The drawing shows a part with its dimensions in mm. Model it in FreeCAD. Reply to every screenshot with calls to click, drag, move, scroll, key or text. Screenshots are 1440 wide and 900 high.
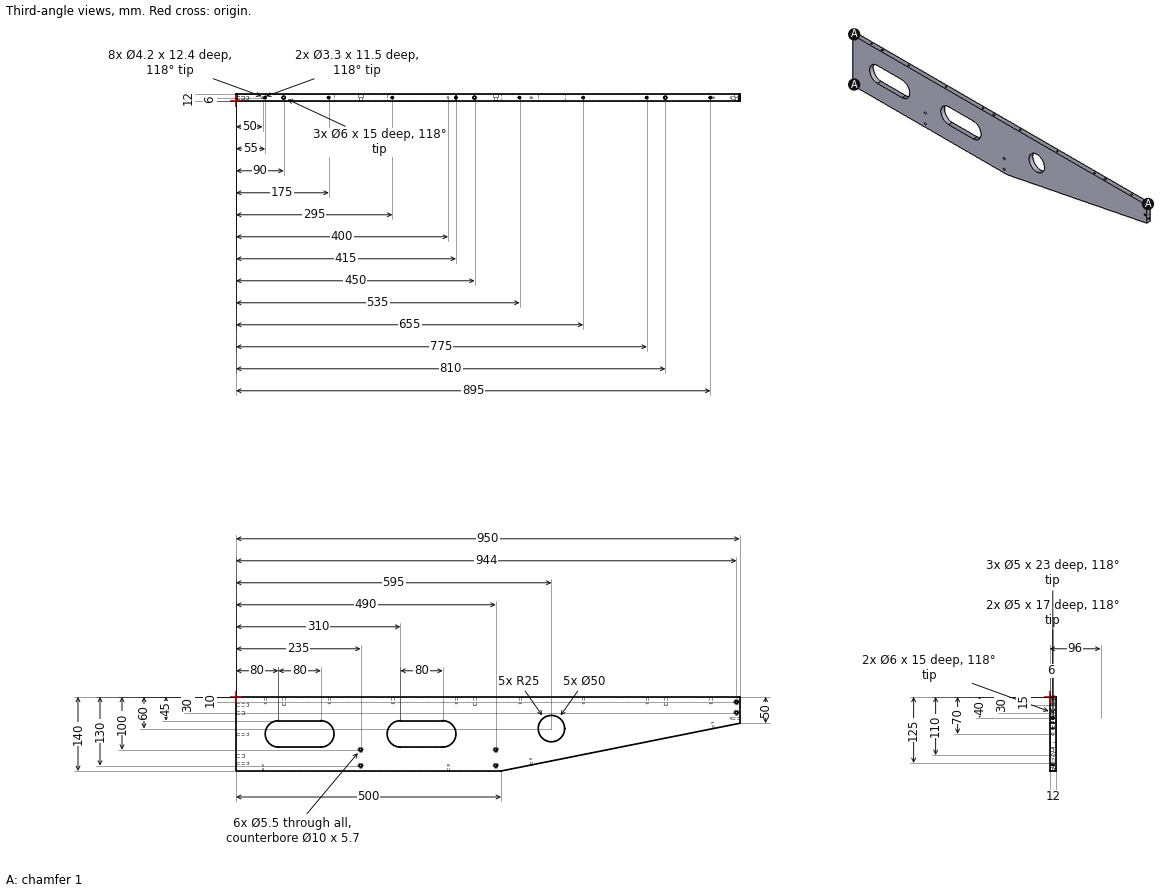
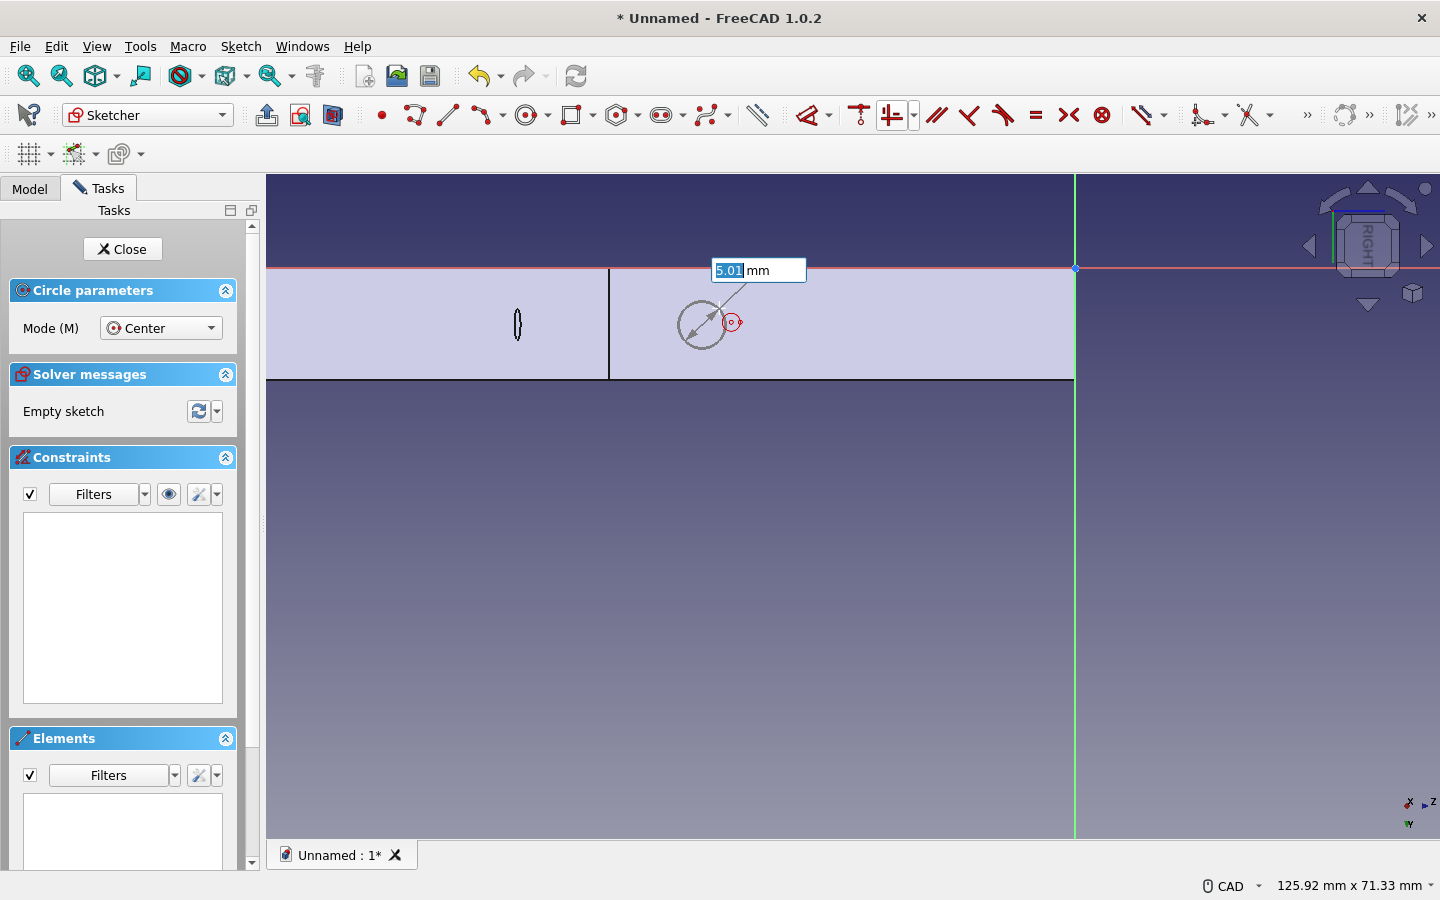
text(5)
key(Return)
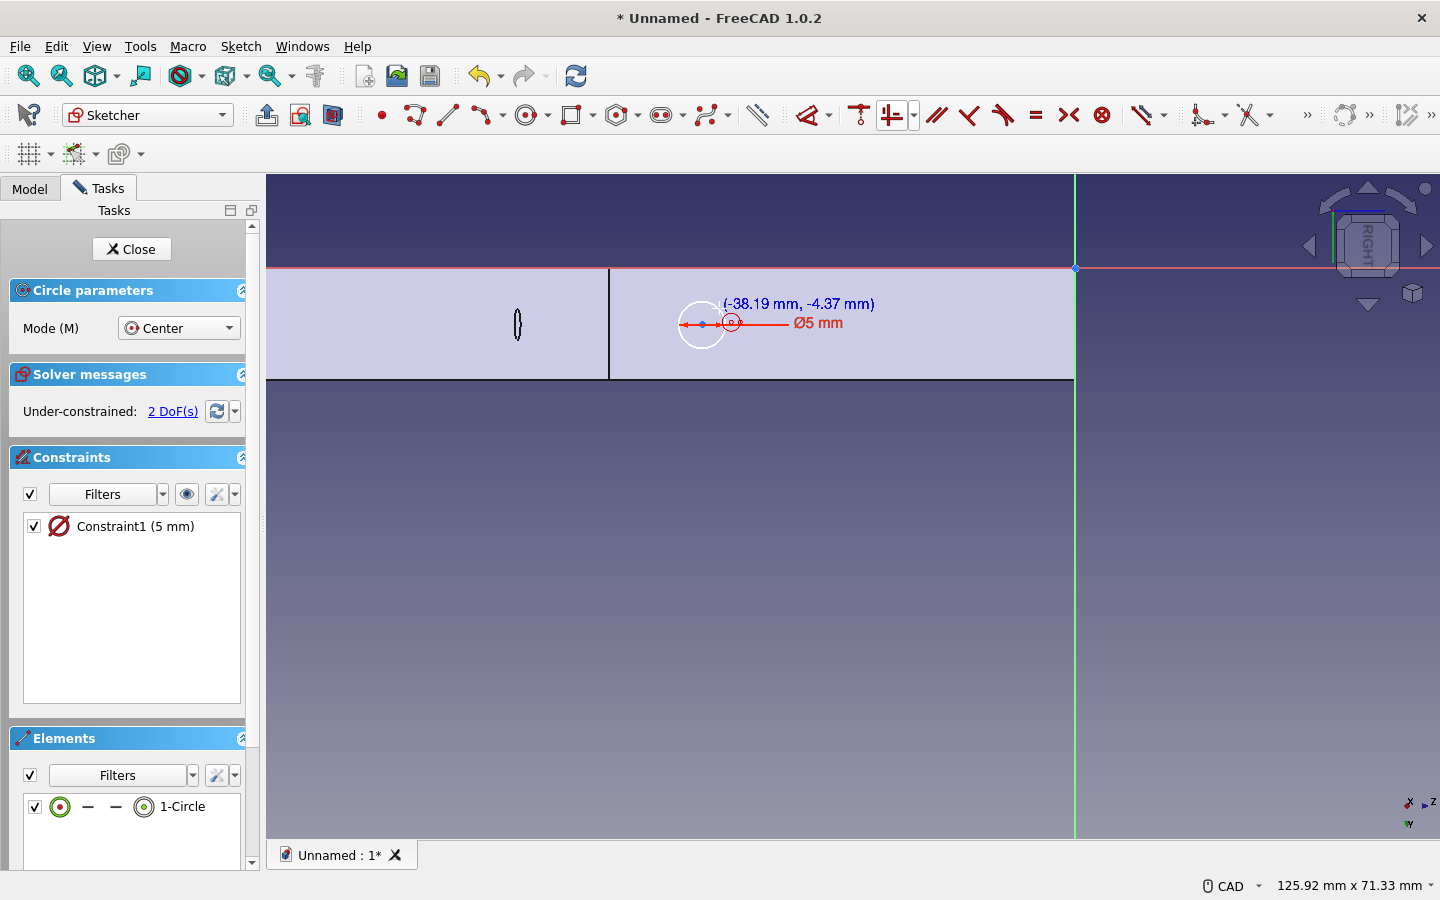
scroll(709, 326, down, 4)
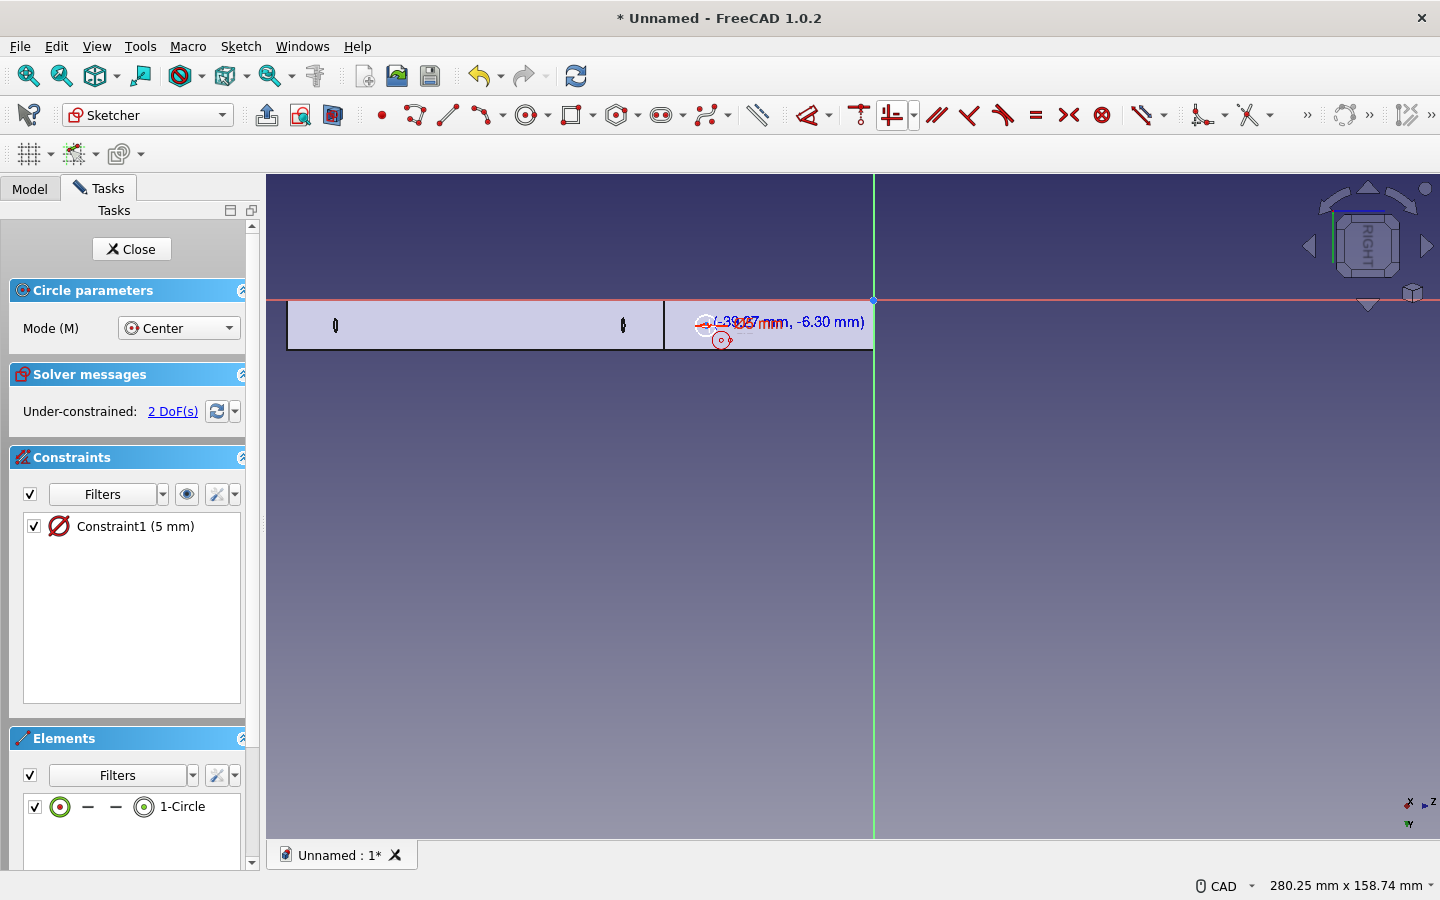
scroll(706, 702, up, 4)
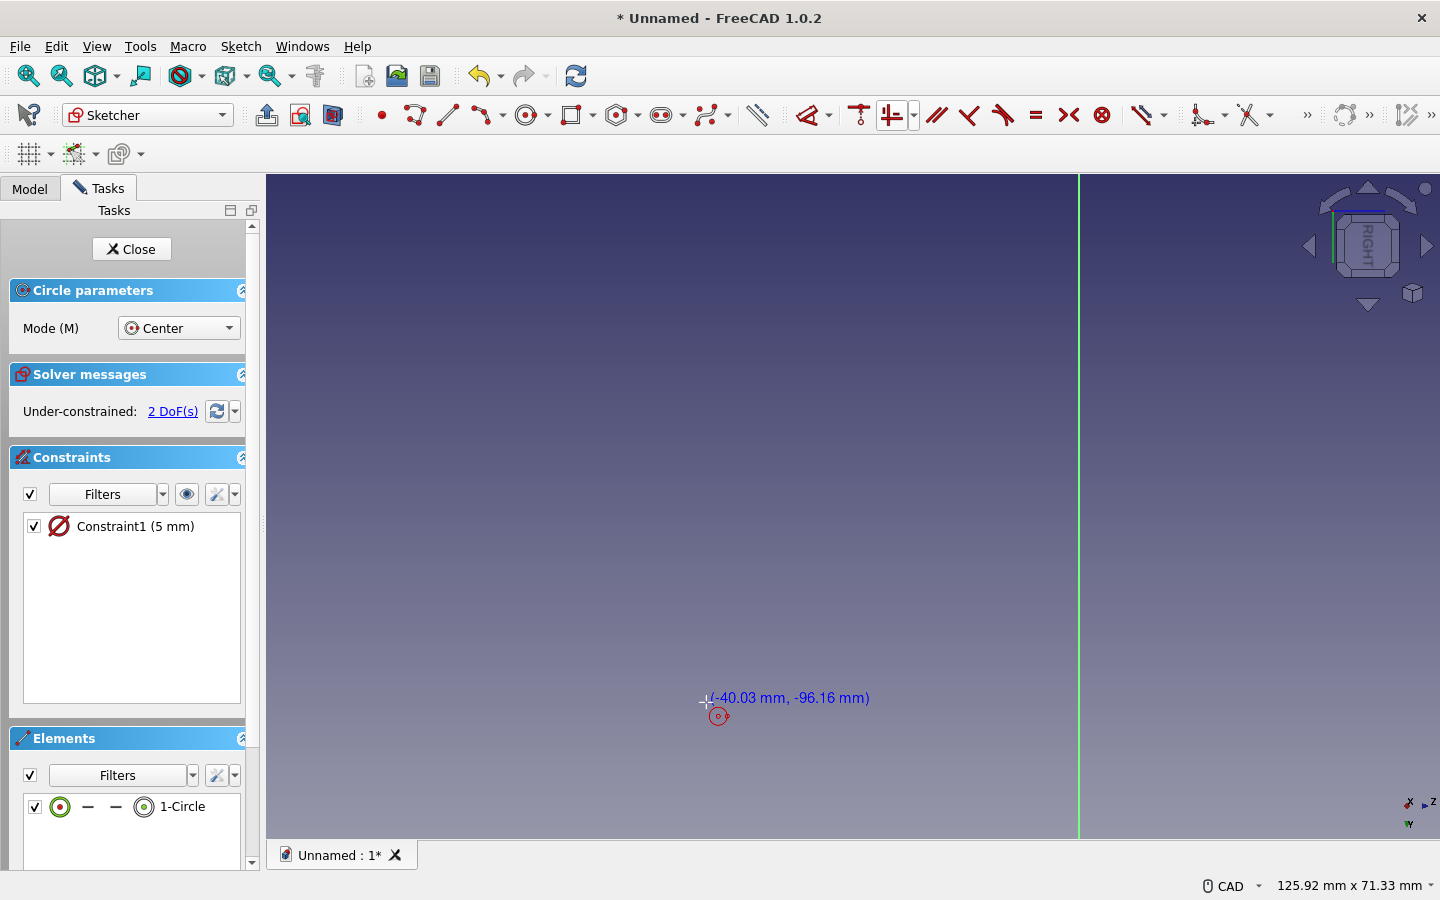
click(706, 702)
move(722, 685)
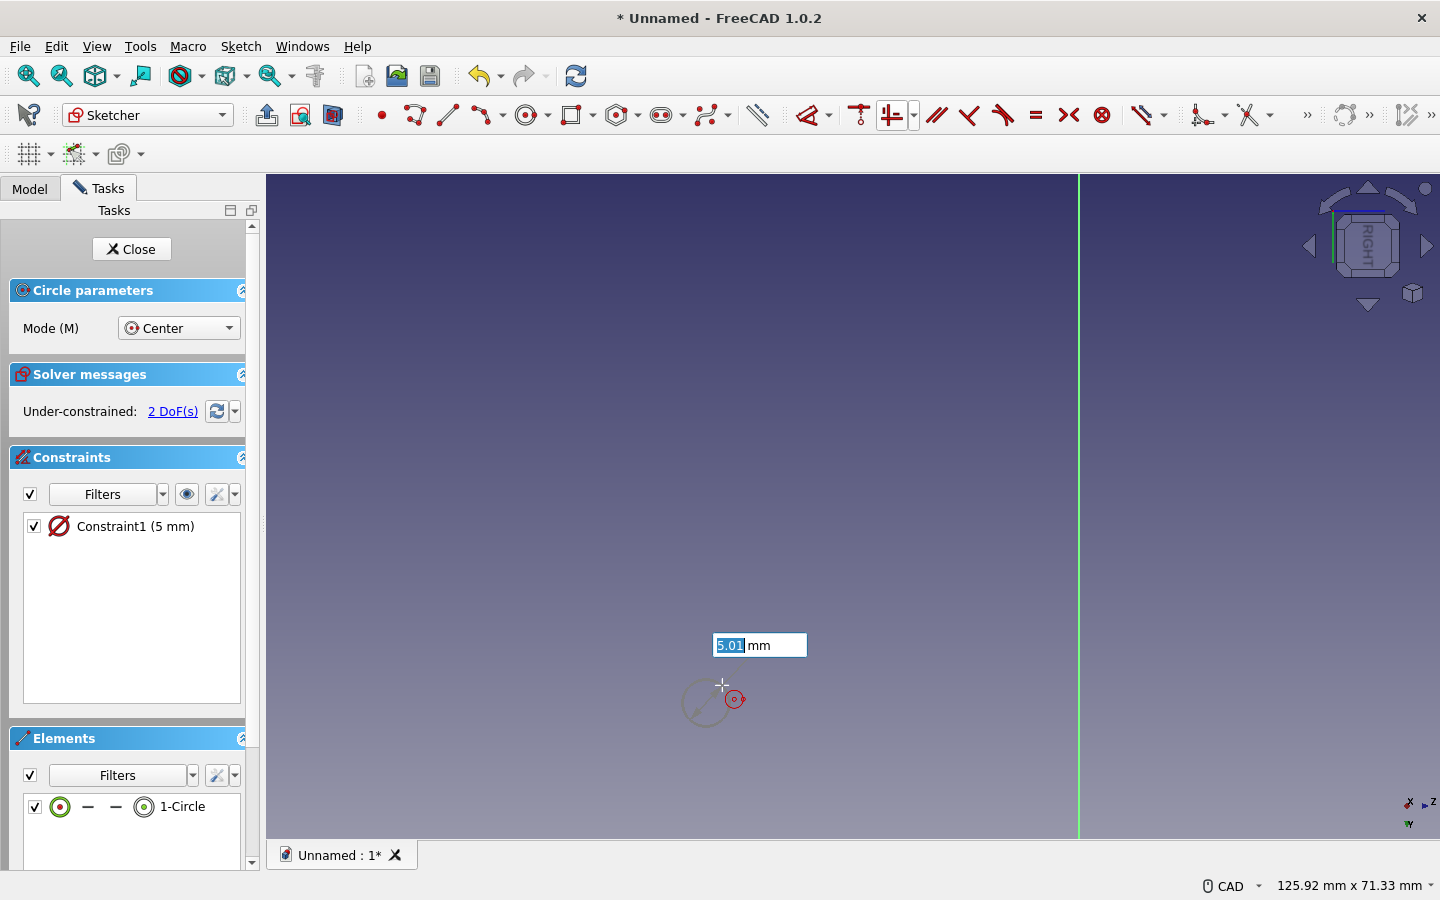
text(5)
key(Return)
key(Escape)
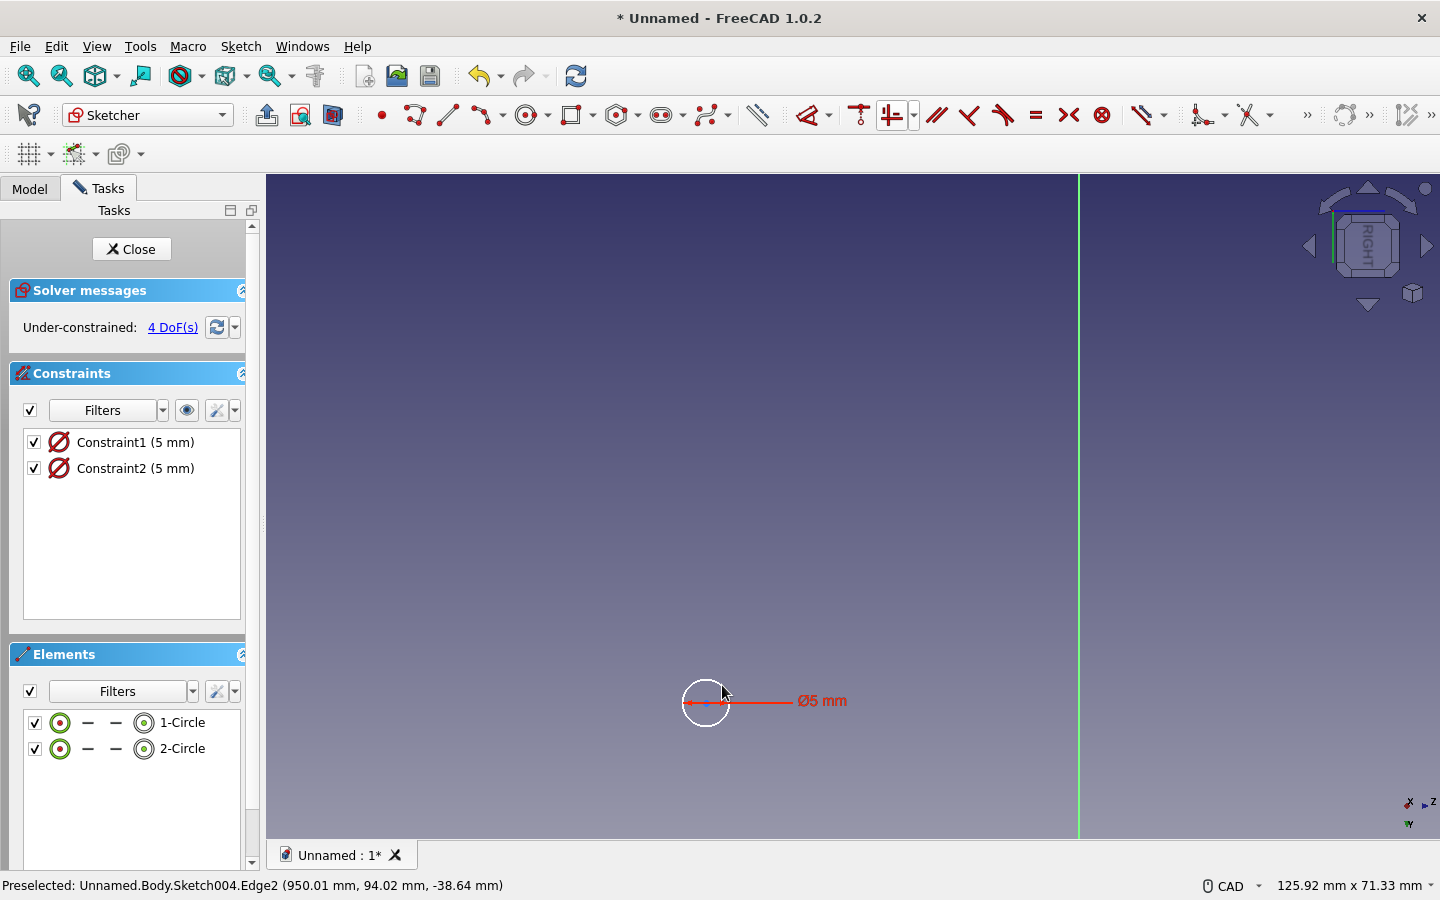
click(806, 116)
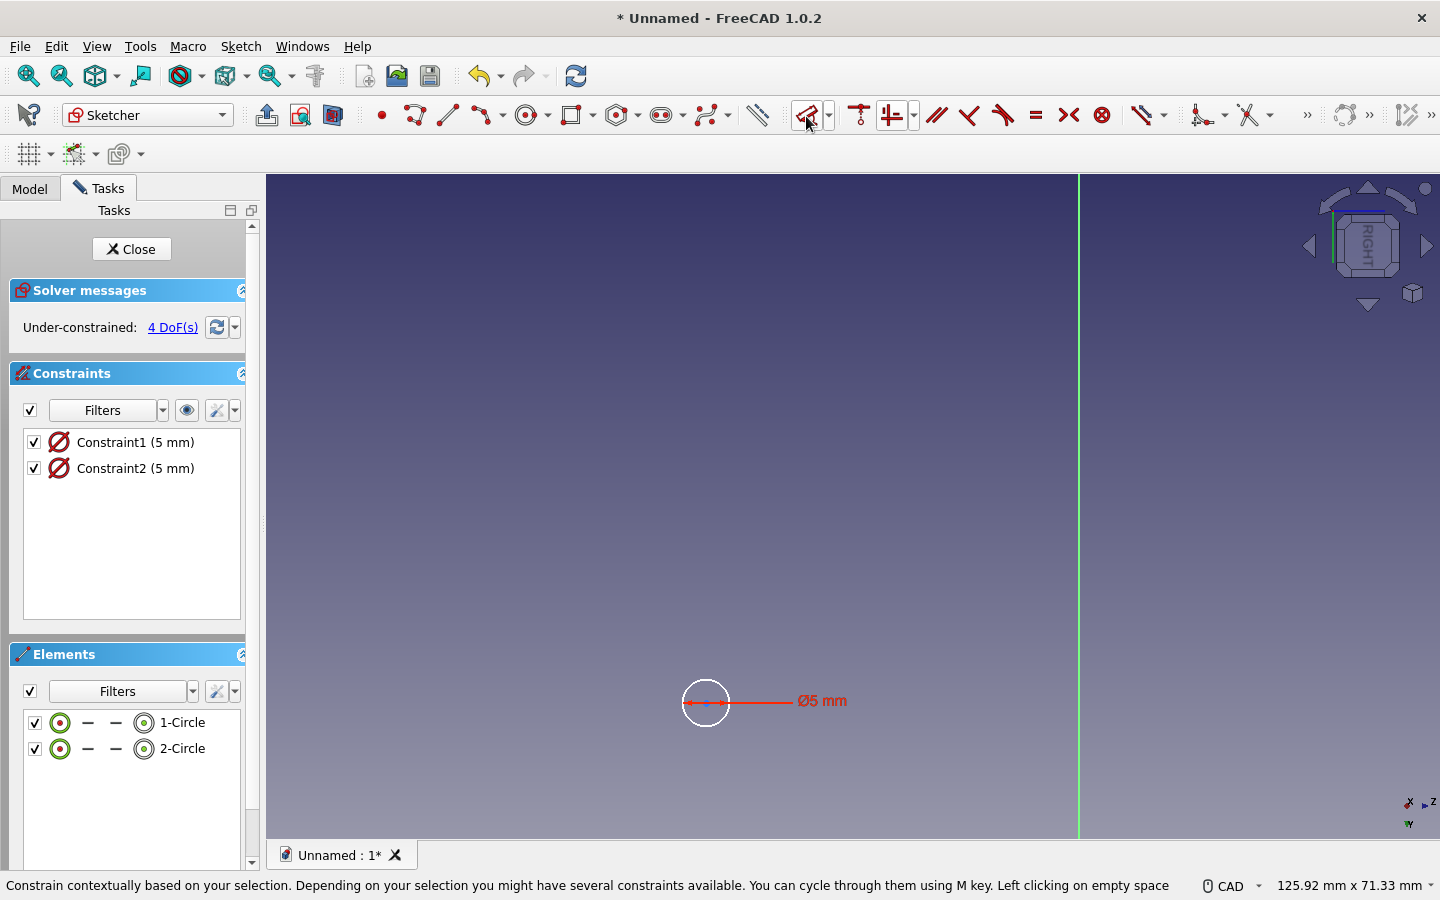
scroll(706, 703, down, 4)